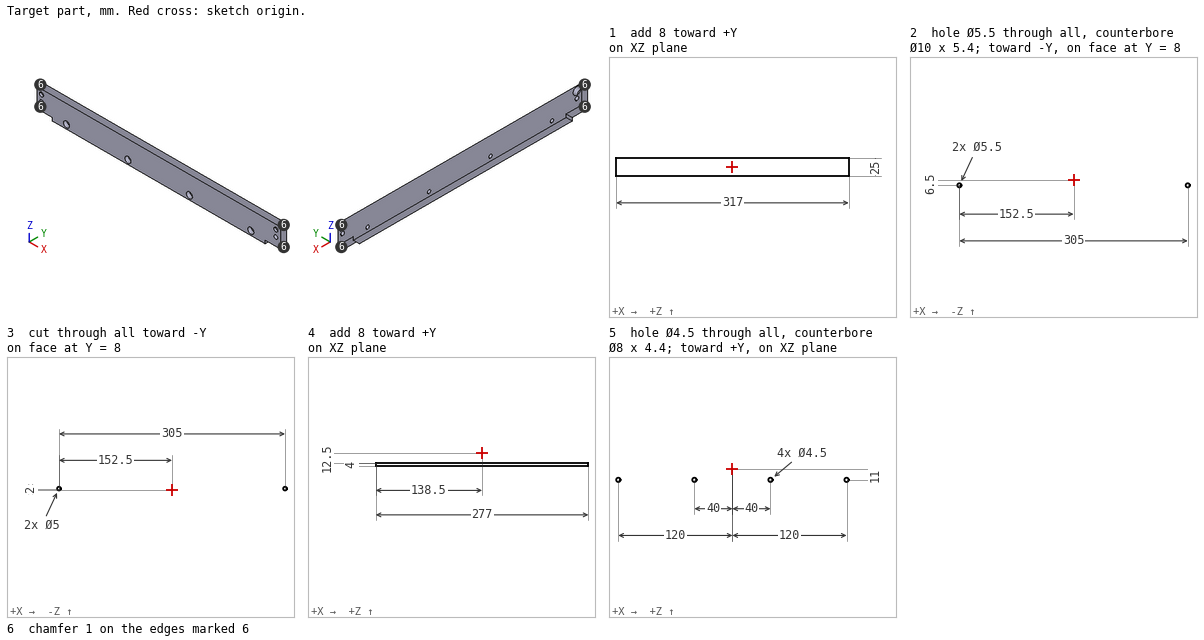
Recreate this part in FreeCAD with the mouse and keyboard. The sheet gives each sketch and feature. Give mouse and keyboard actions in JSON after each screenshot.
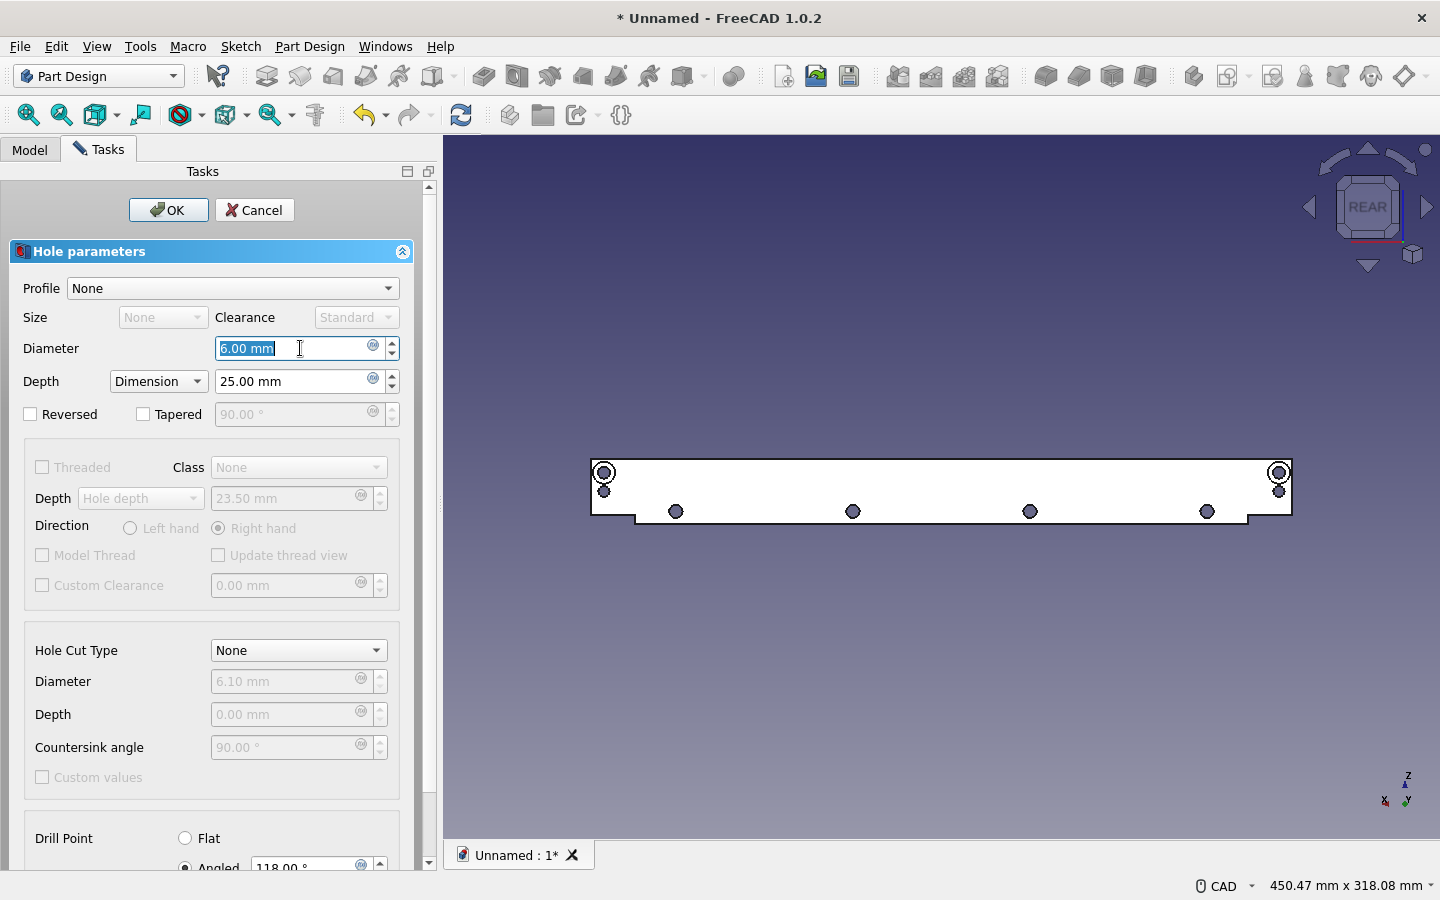
{"action": "type", "text": "4.5"}
{"action": "key", "text": "Tab"}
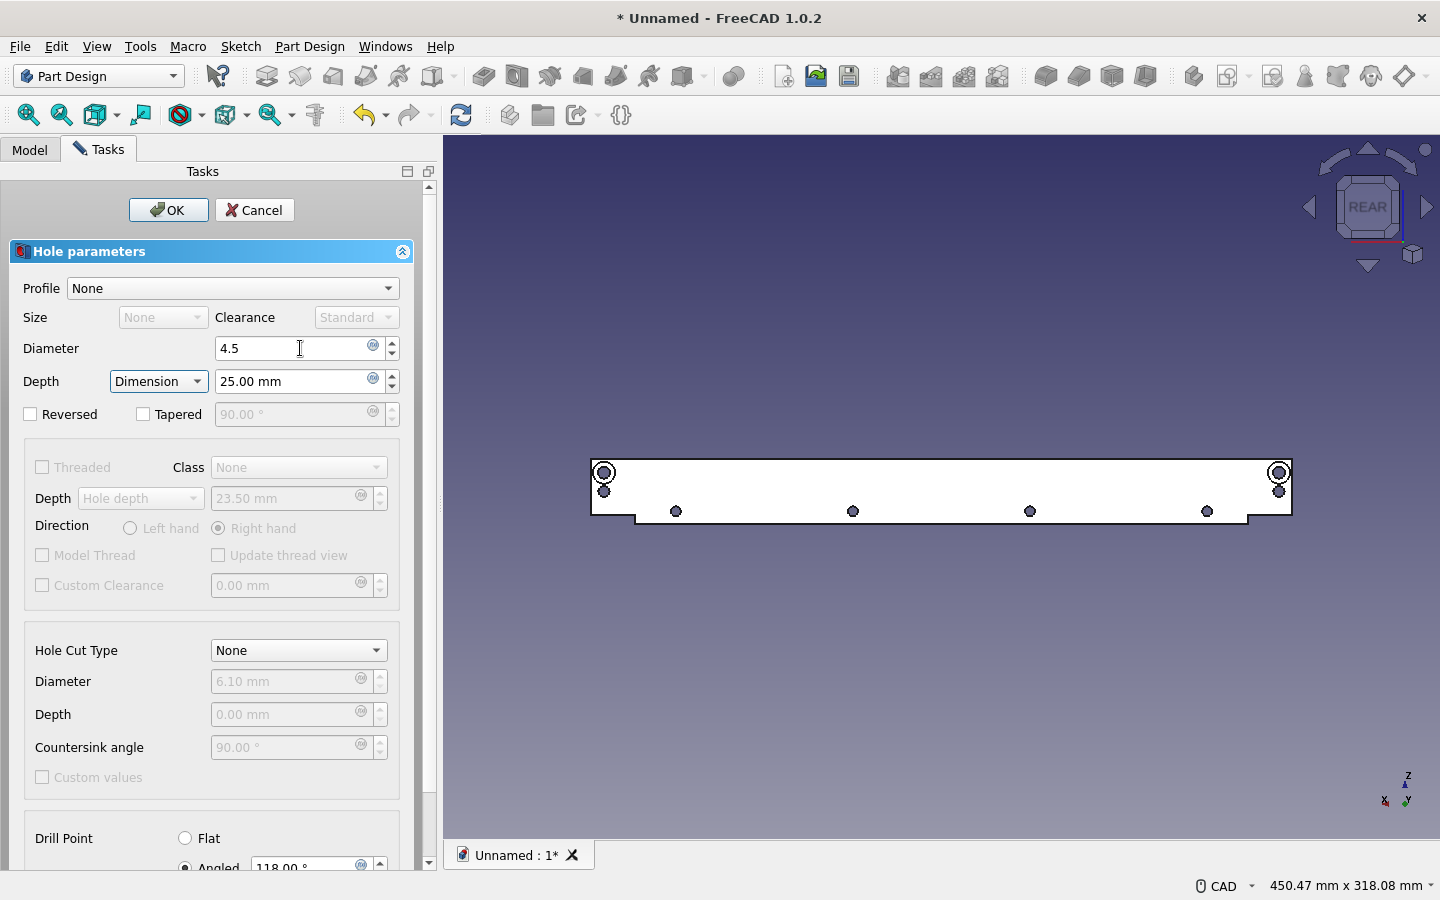
{"action": "left_click", "coordinate": [160, 382]}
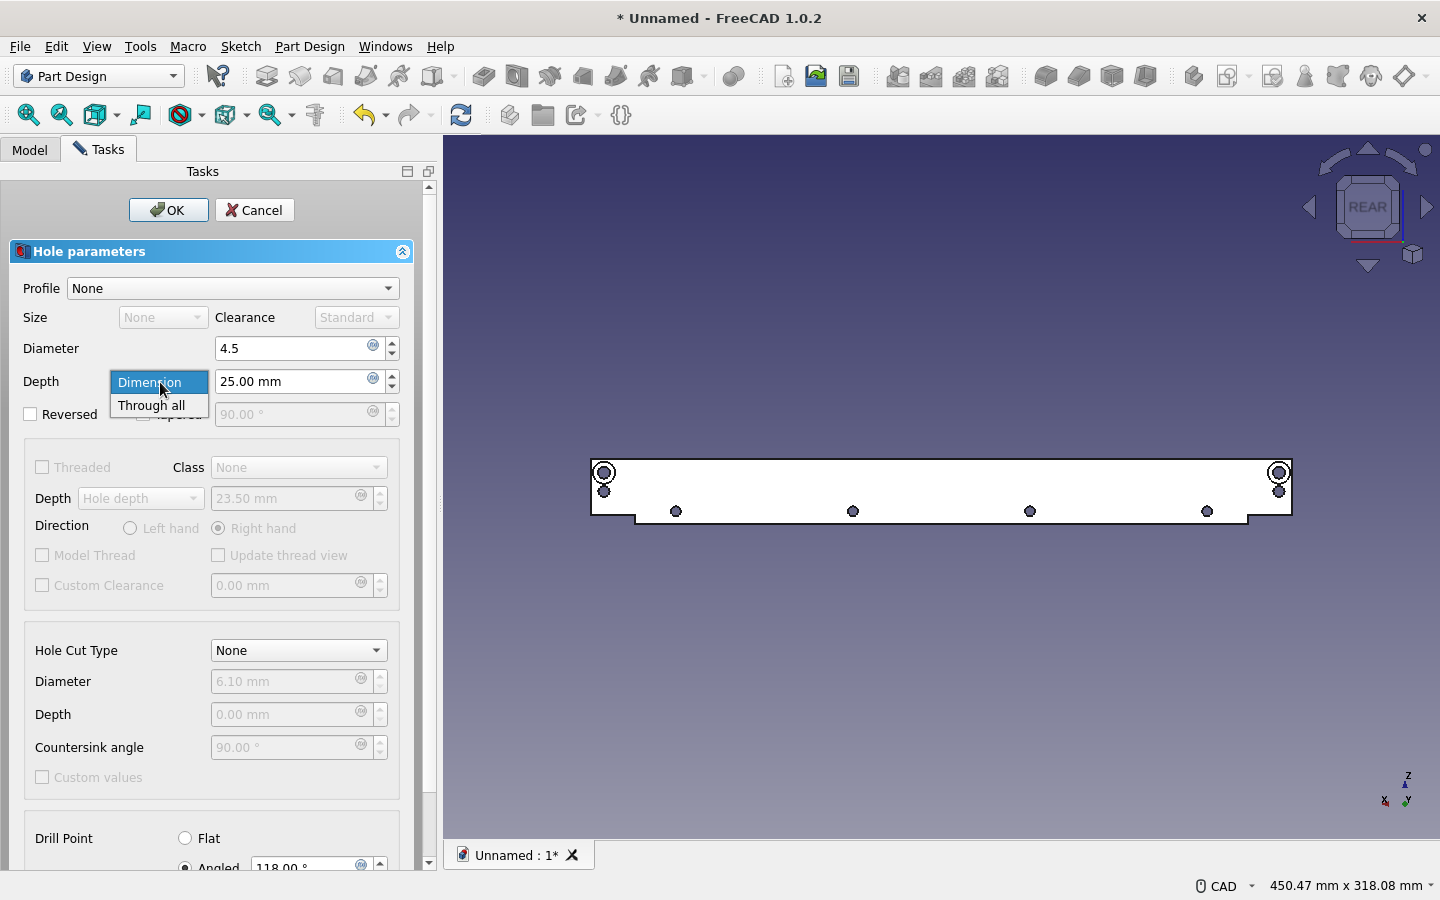
{"action": "left_click", "coordinate": [158, 406]}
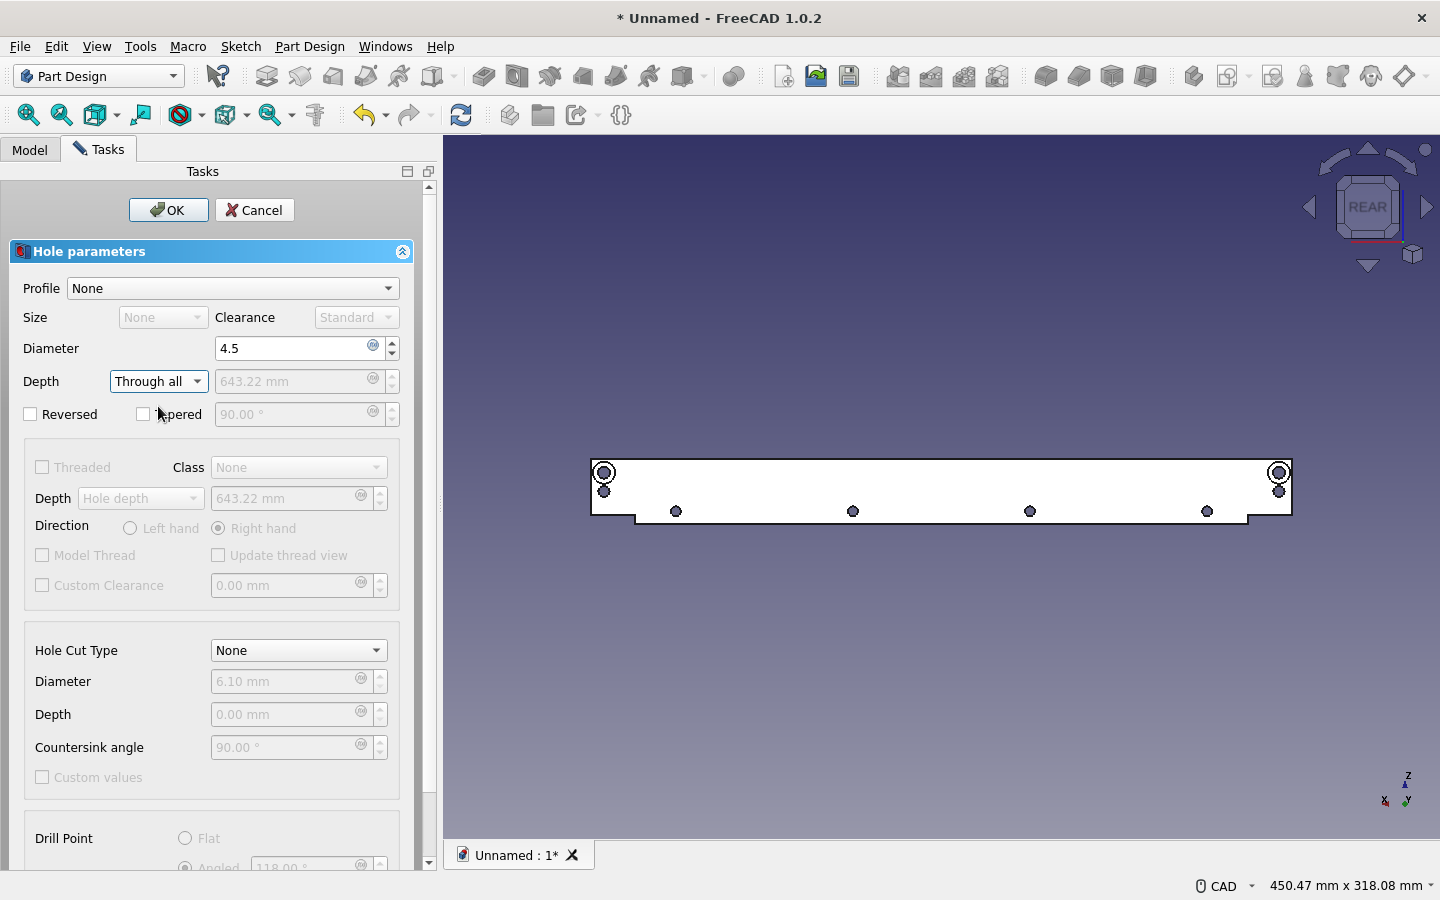
{"action": "left_click", "coordinate": [300, 650]}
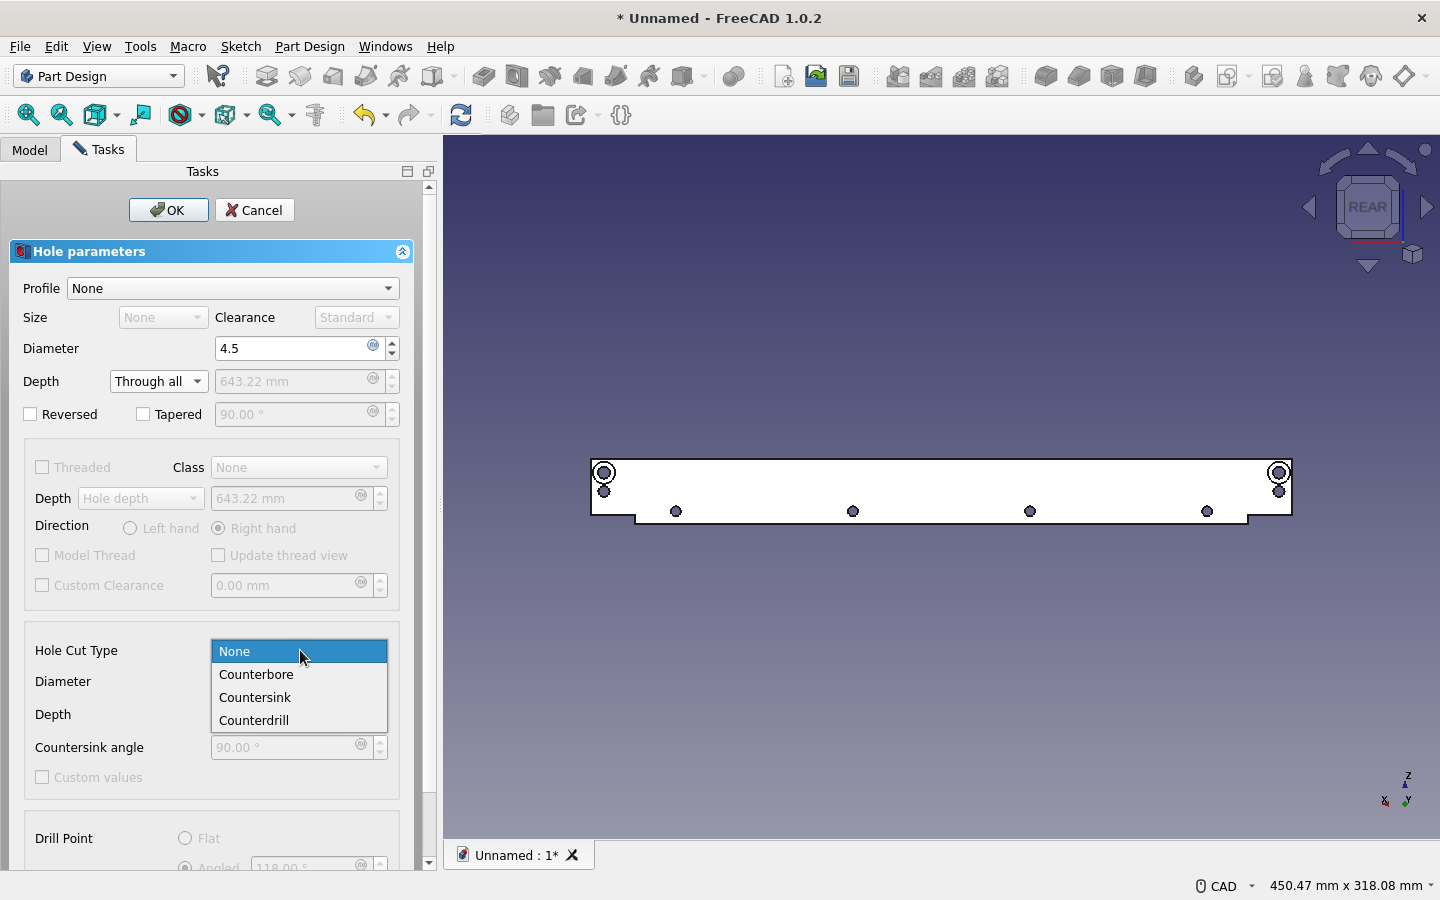
{"action": "left_click", "coordinate": [298, 674]}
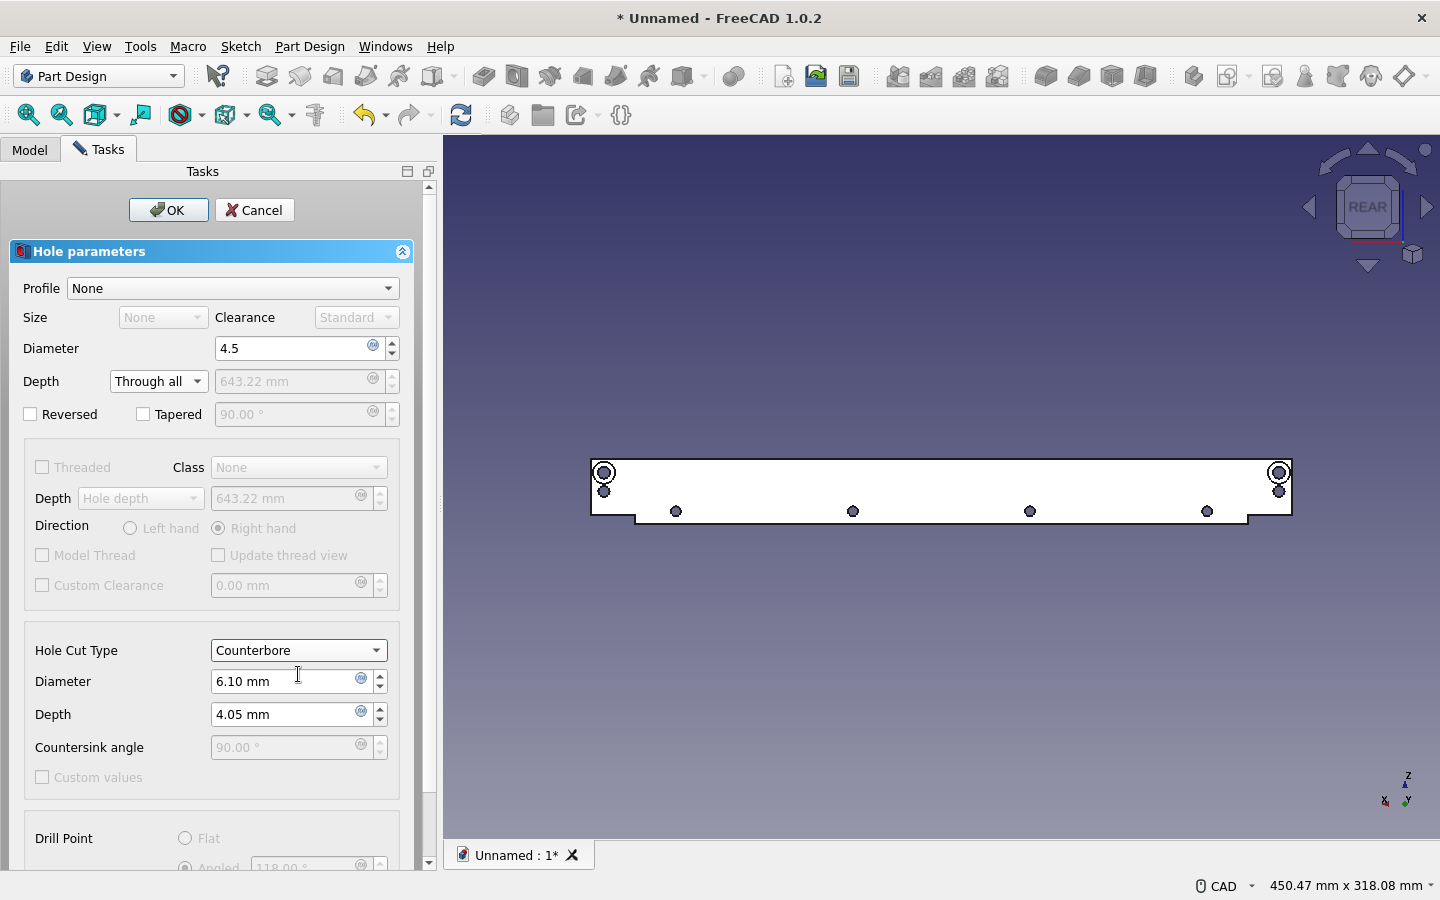
{"action": "triple_click", "coordinate": [292, 682]}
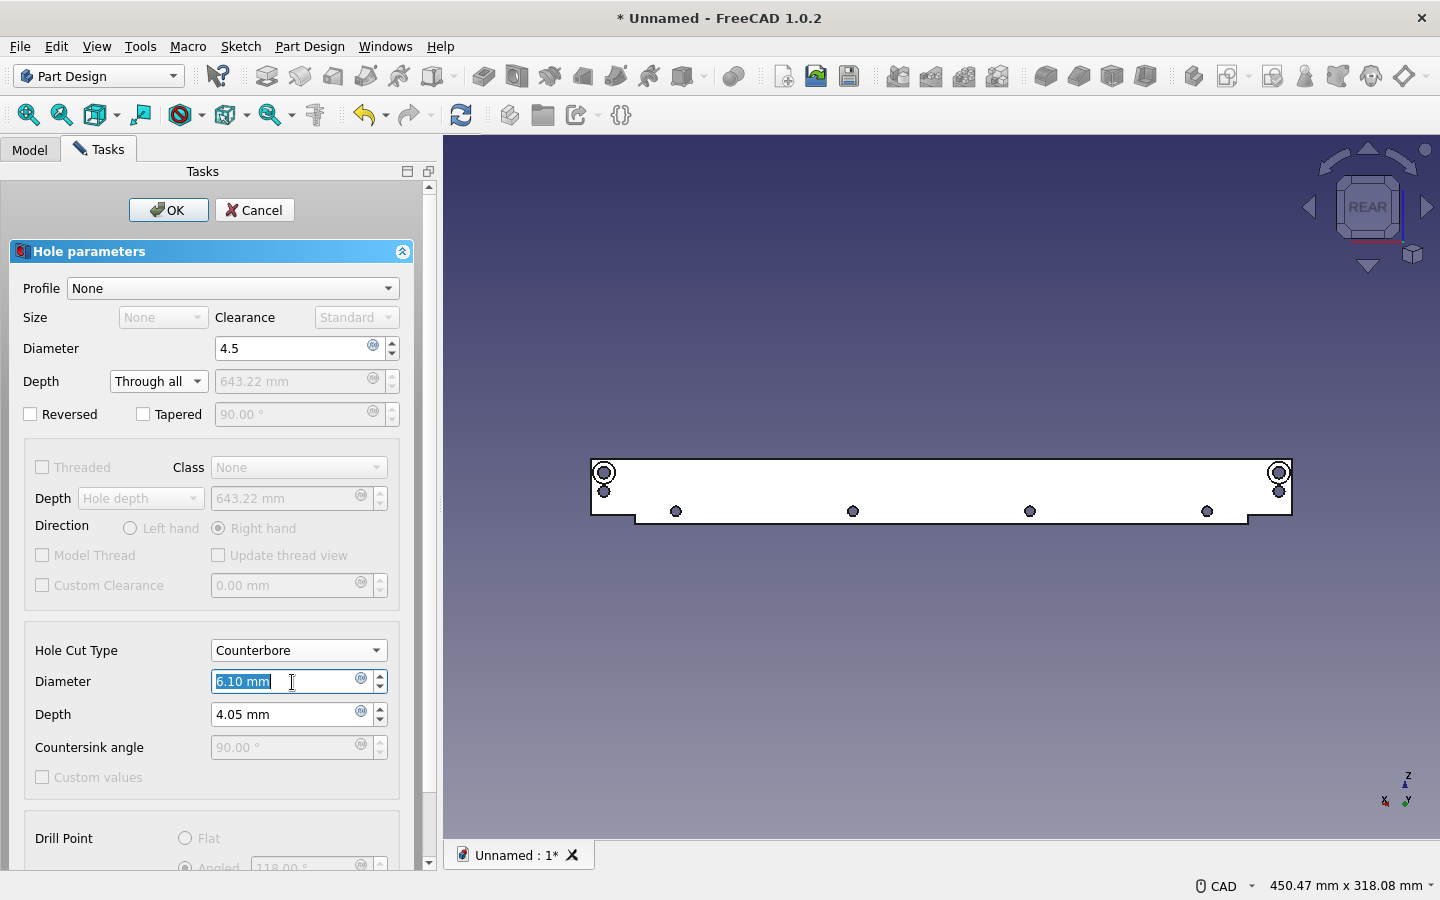
{"action": "type", "text": "8"}
{"action": "key", "text": "Tab"}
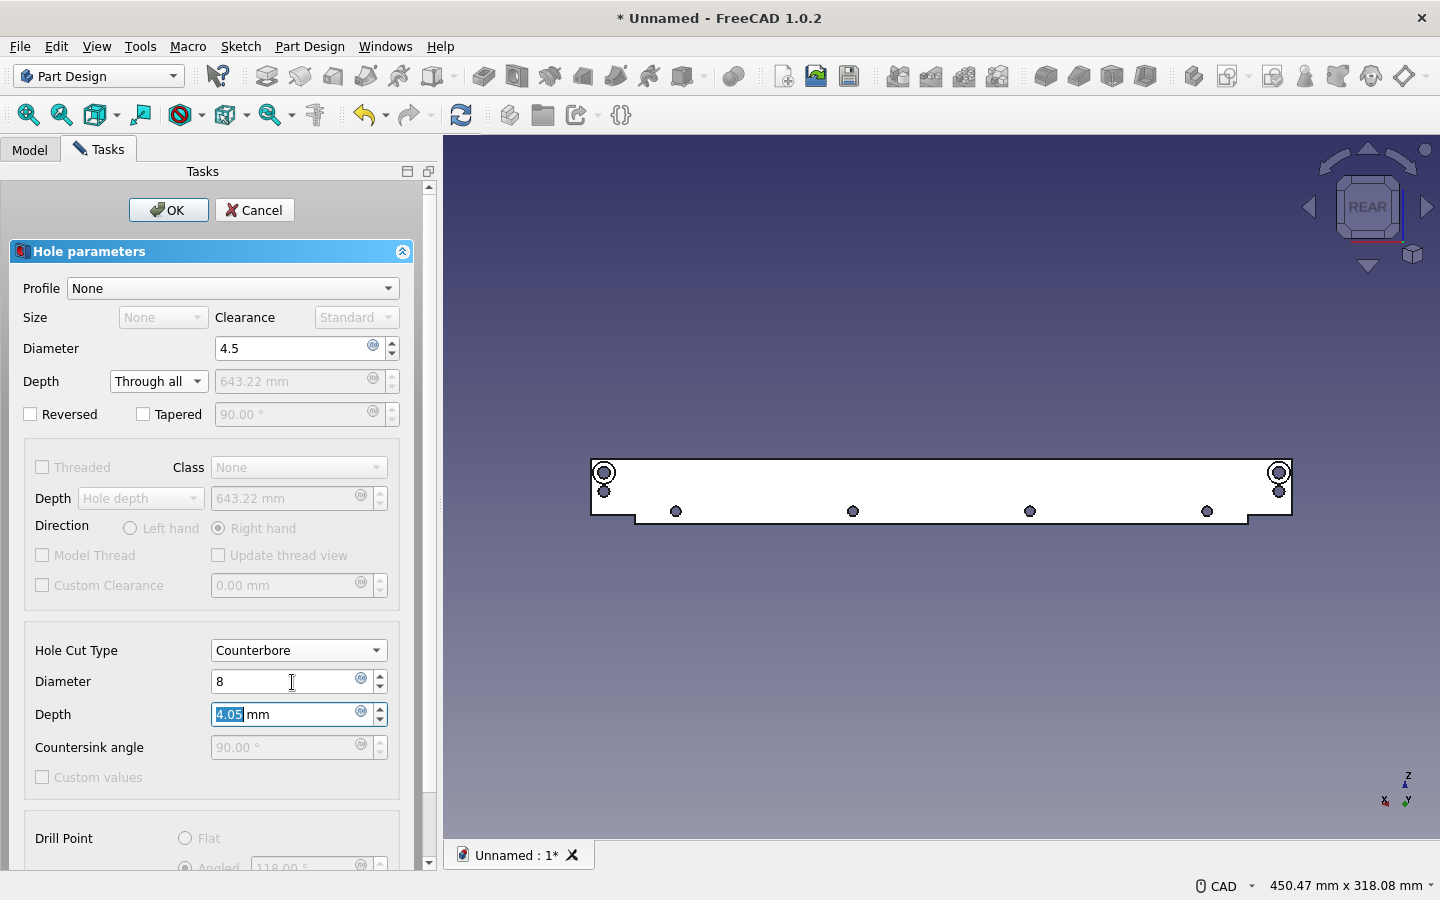
{"action": "type", "text": "4.4"}
{"action": "key", "text": "Tab"}